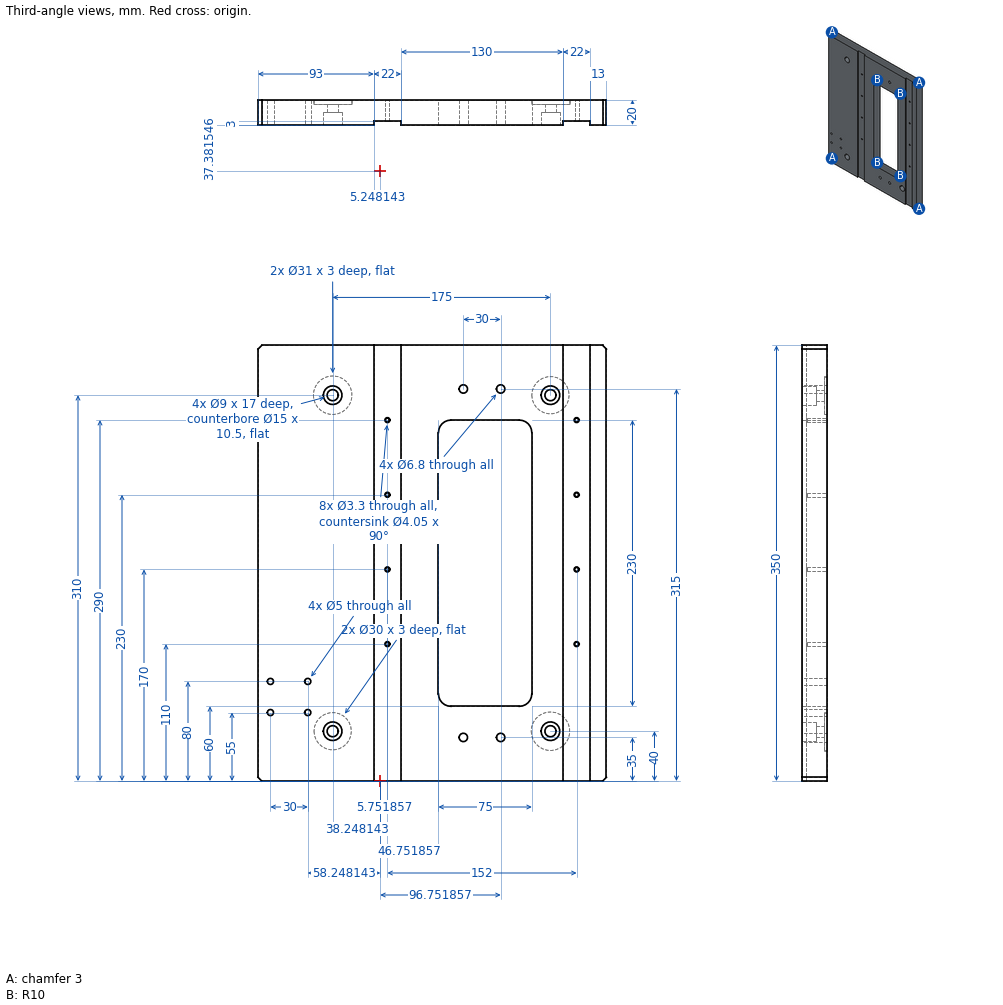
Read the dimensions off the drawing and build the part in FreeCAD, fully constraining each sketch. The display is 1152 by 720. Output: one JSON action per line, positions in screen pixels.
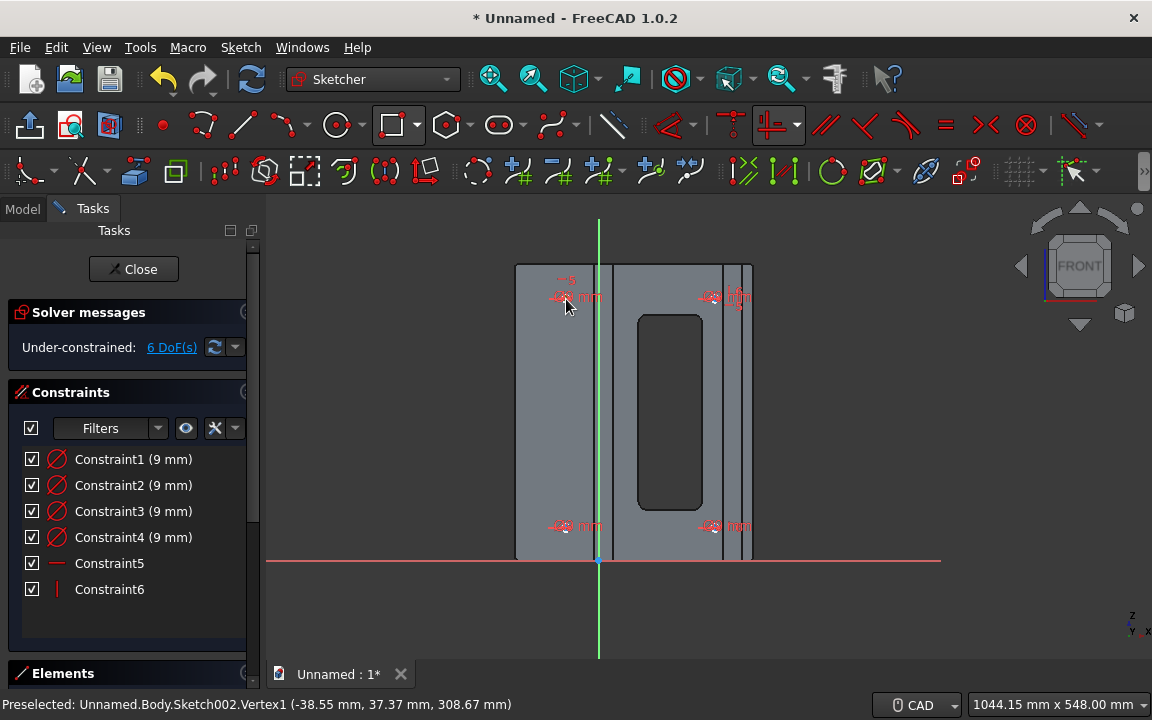
{"action": "left_click", "coordinate": [566, 528]}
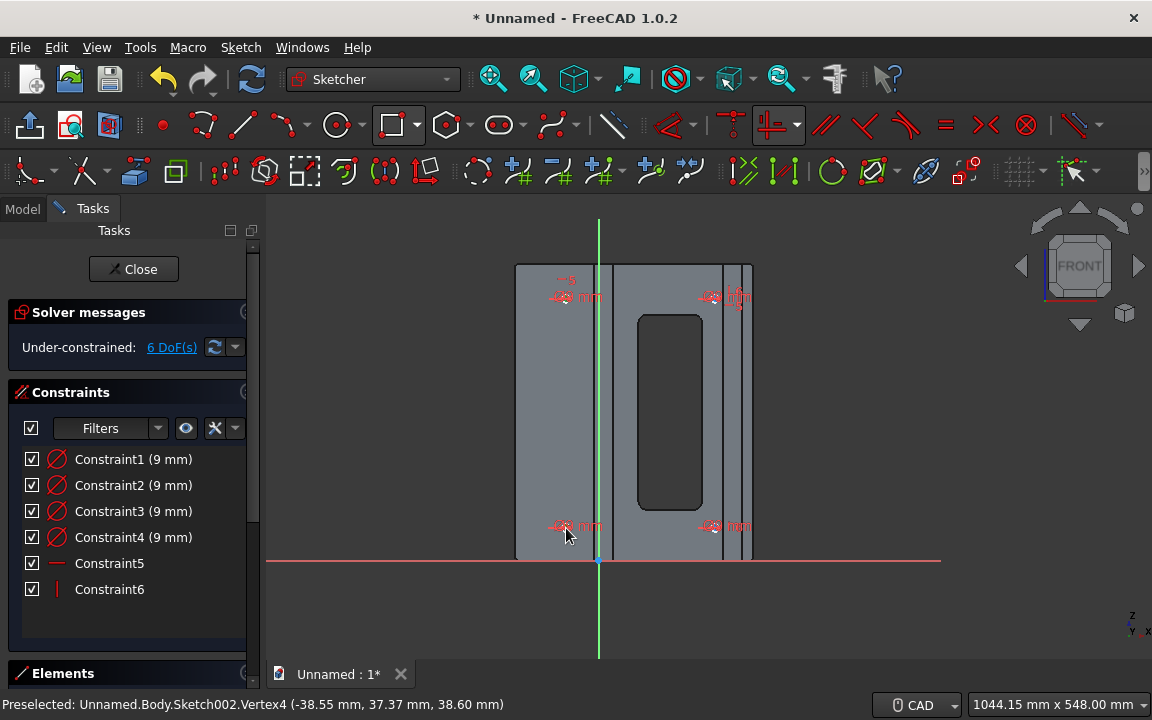
{"action": "left_click", "coordinate": [800, 126]}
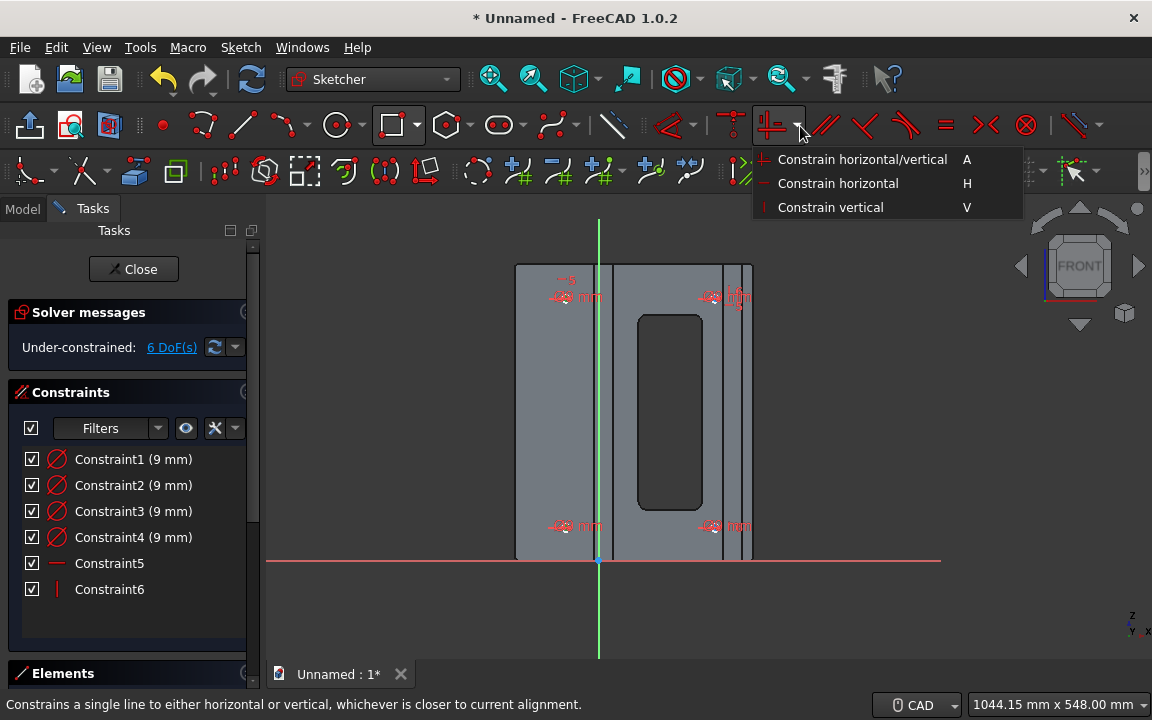
{"action": "left_click", "coordinate": [888, 207]}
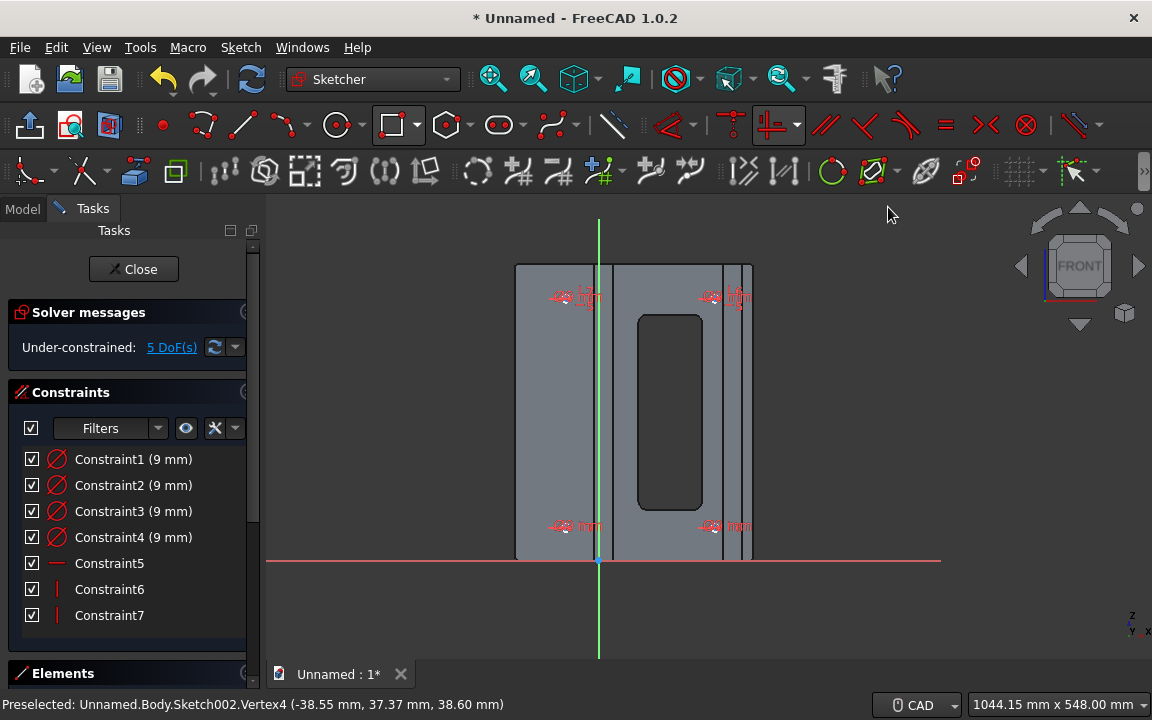
{"action": "left_click", "coordinate": [715, 528]}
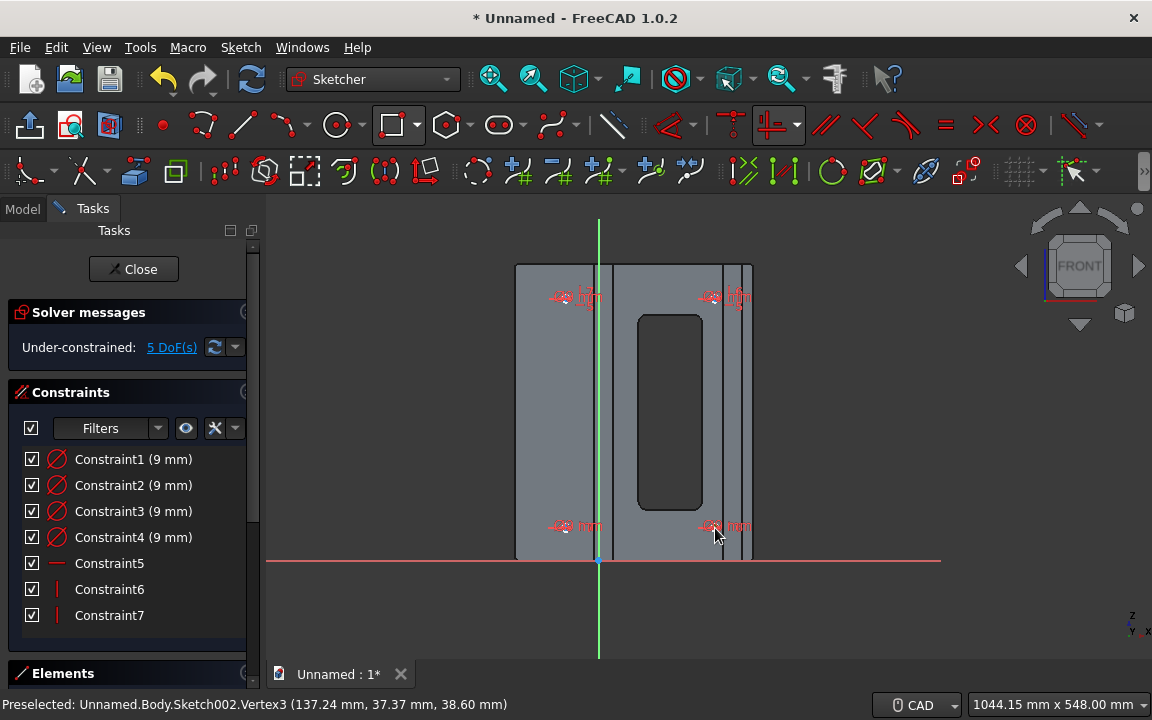
{"action": "left_click", "coordinate": [566, 528]}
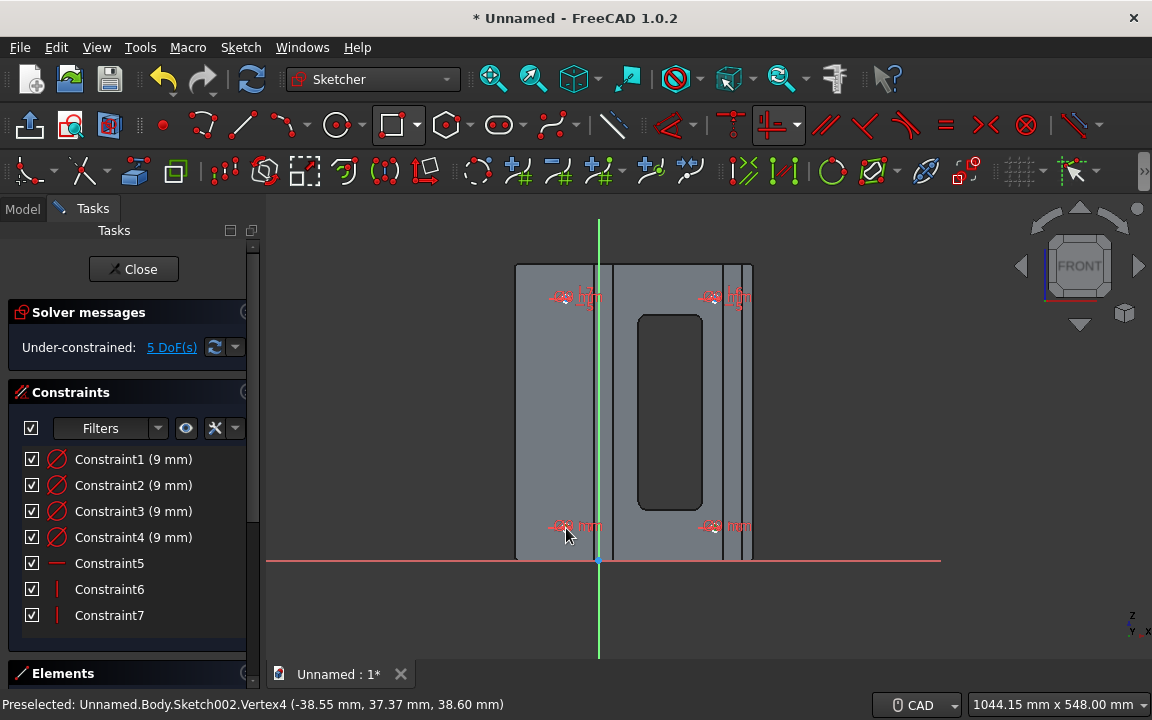
{"action": "left_click", "coordinate": [800, 126]}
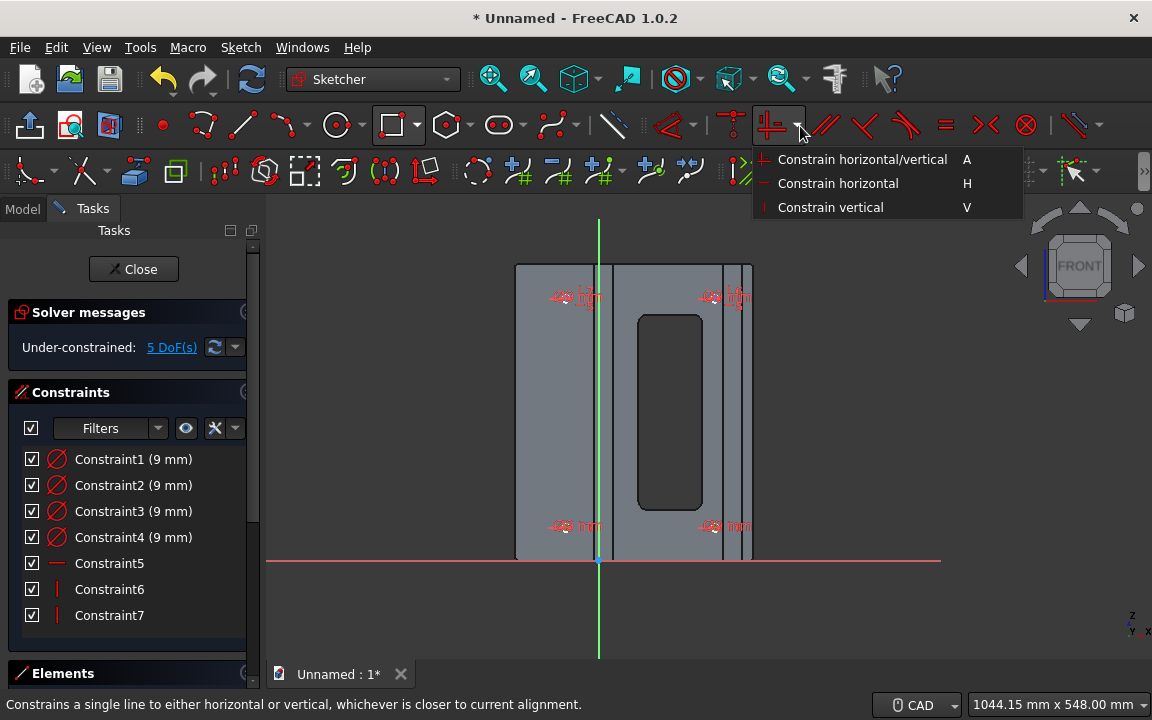
{"action": "left_click", "coordinate": [888, 183]}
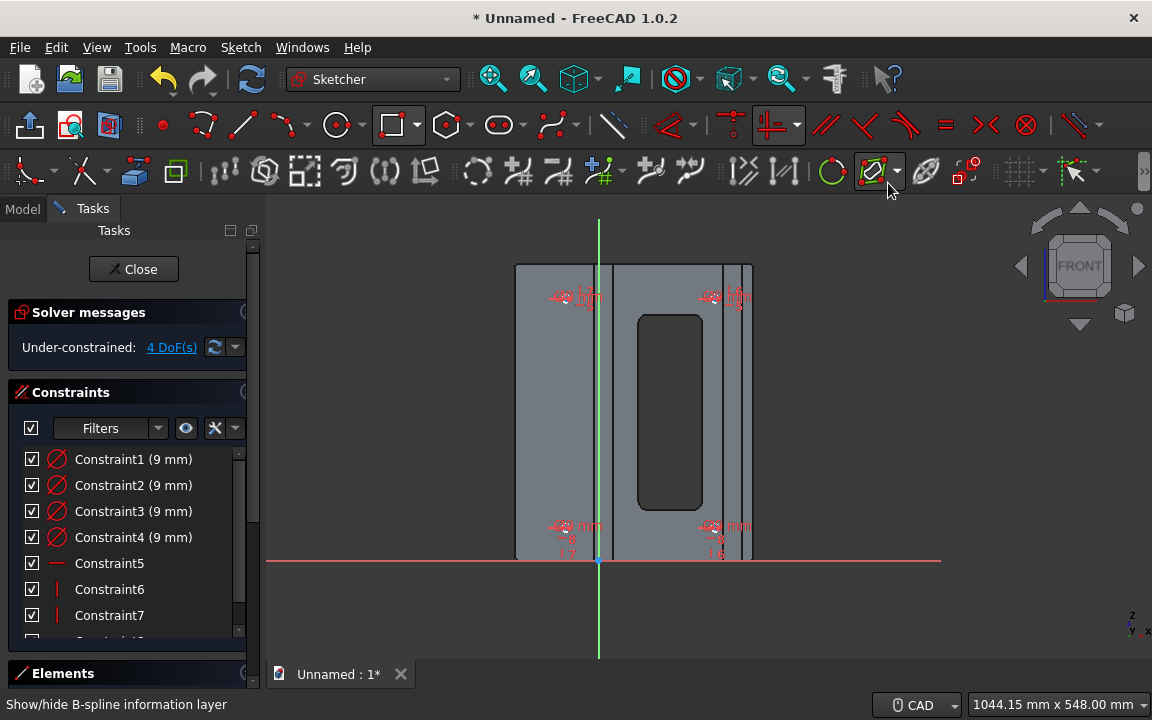
{"action": "left_click", "coordinate": [668, 126]}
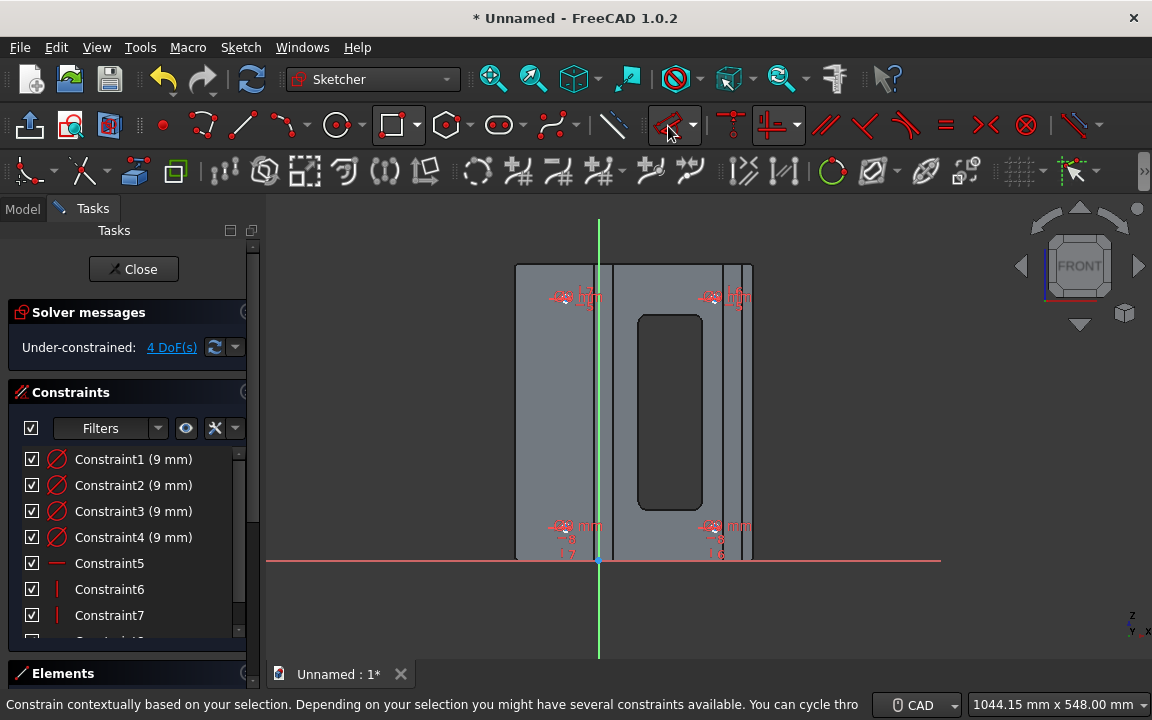
{"action": "left_click", "coordinate": [715, 528]}
{"action": "left_click", "coordinate": [749, 544]}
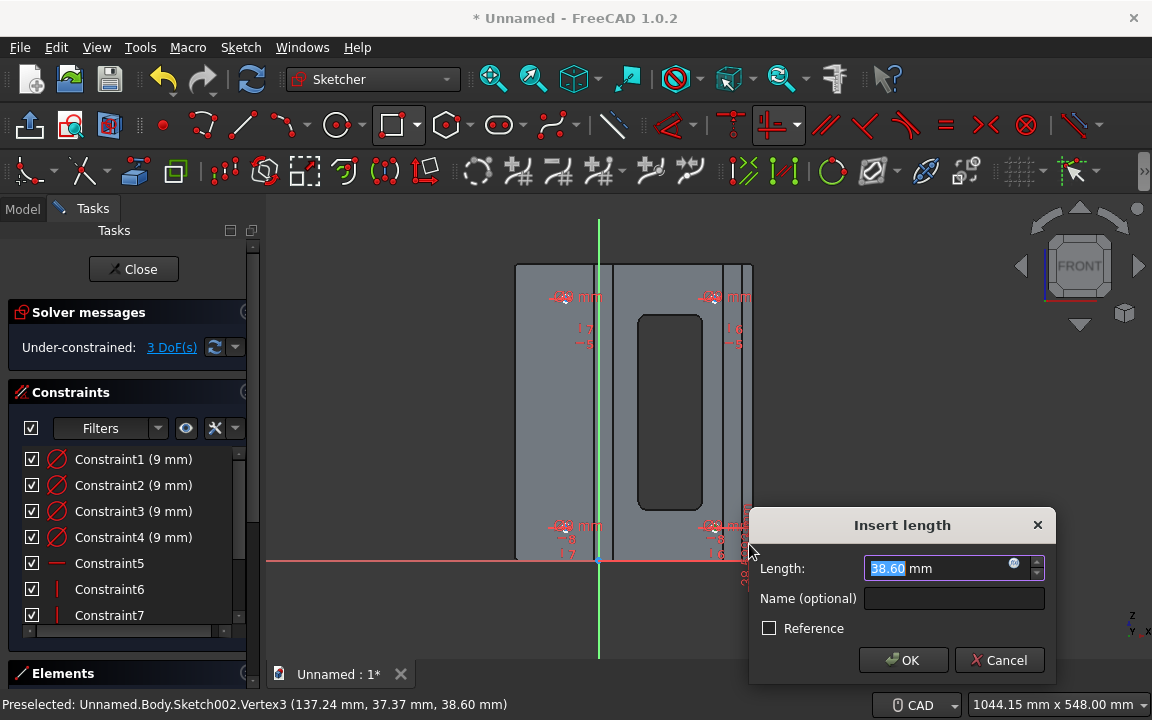
{"action": "type", "text": "40"}
{"action": "key", "text": "Return"}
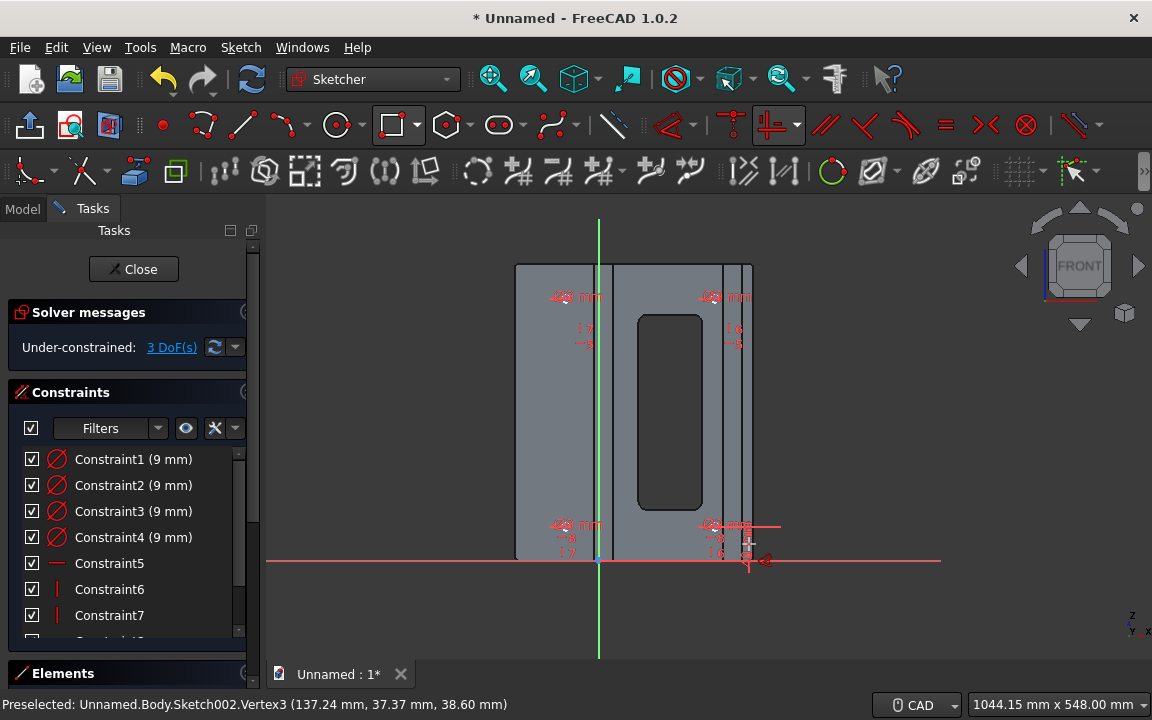
{"action": "left_click", "coordinate": [566, 299]}
{"action": "left_click", "coordinate": [532, 430]}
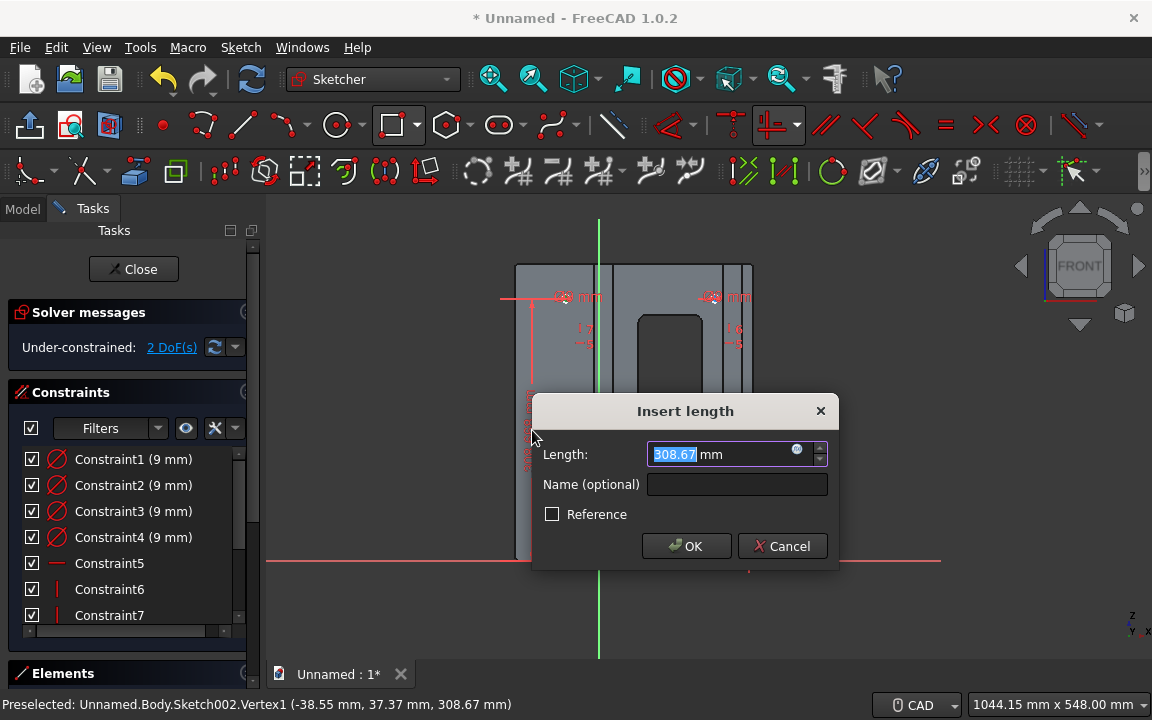
{"action": "type", "text": "310"}
{"action": "key", "text": "Return"}